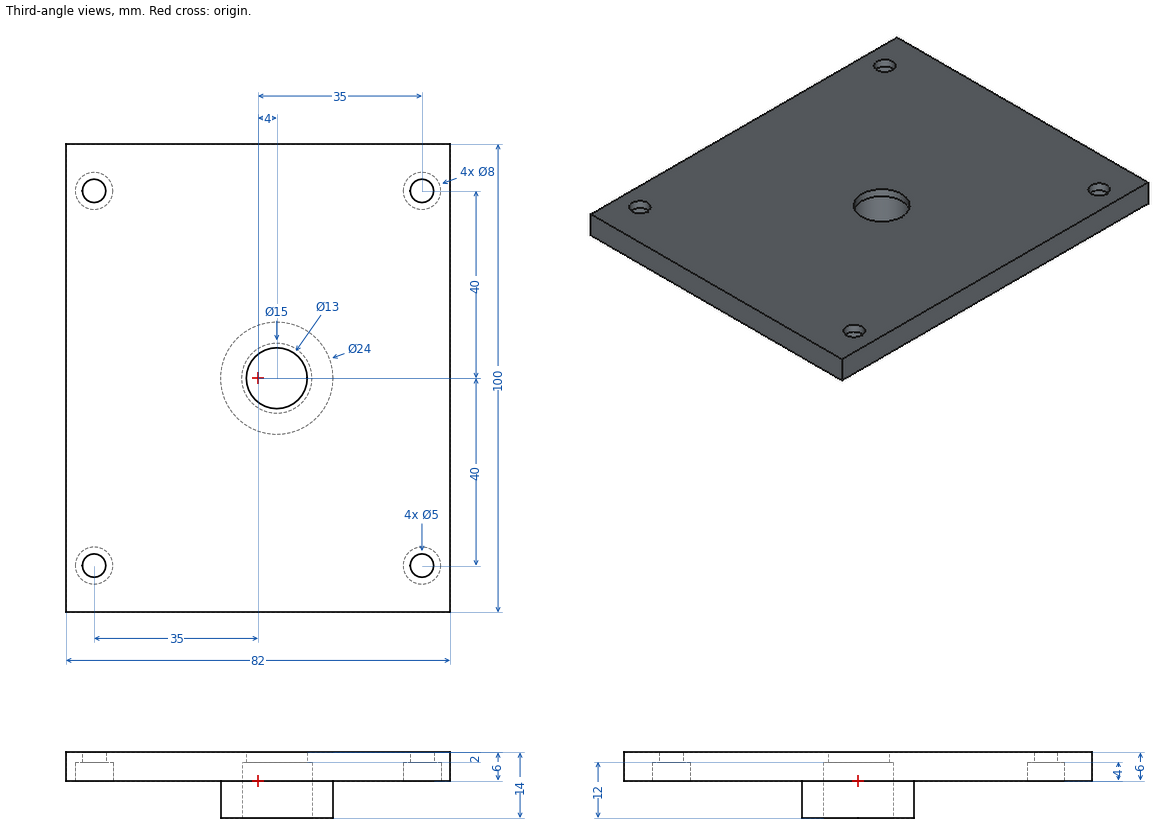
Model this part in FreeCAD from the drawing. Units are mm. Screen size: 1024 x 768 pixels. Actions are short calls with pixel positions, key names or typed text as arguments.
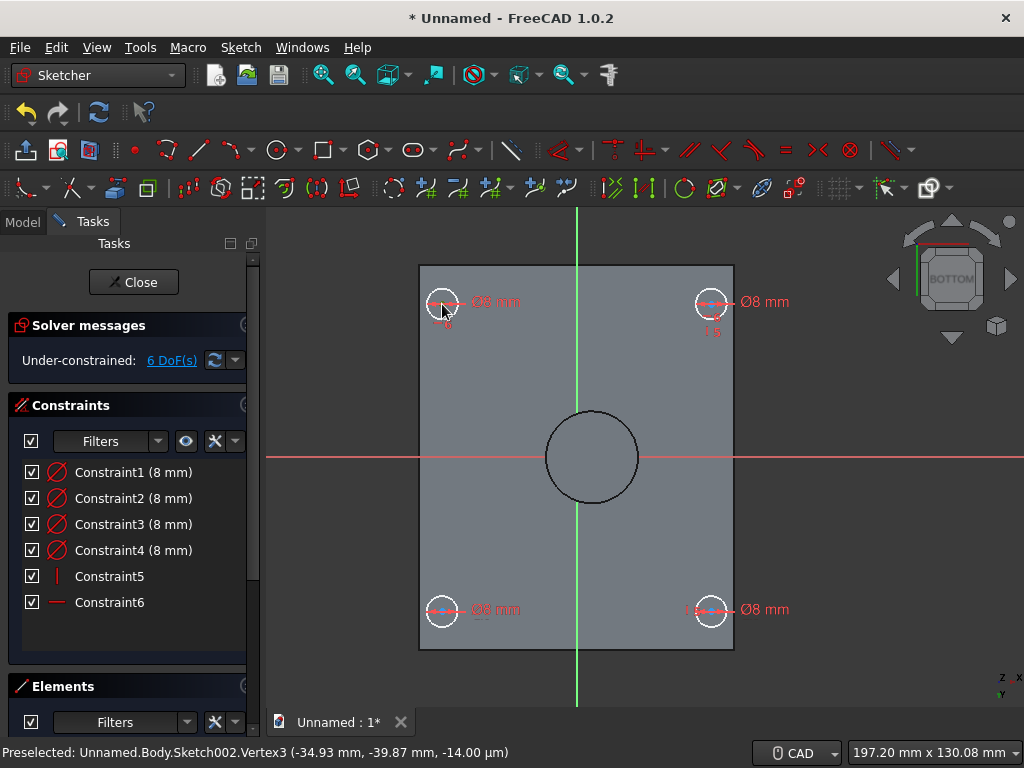
click(442, 612)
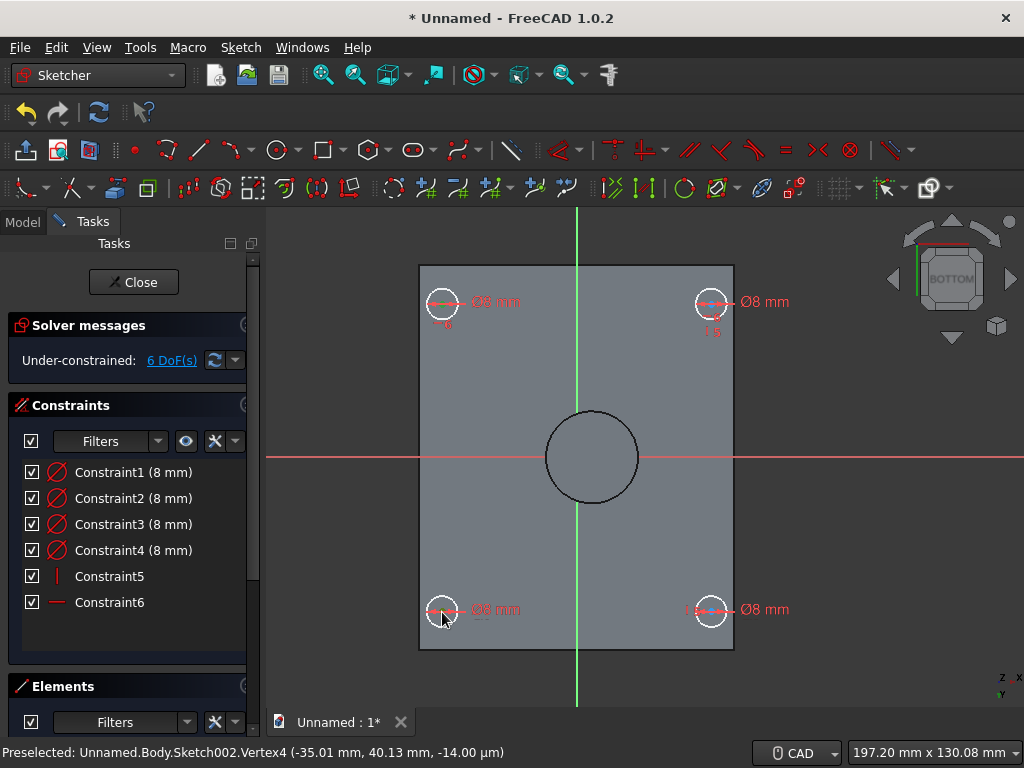
click(668, 150)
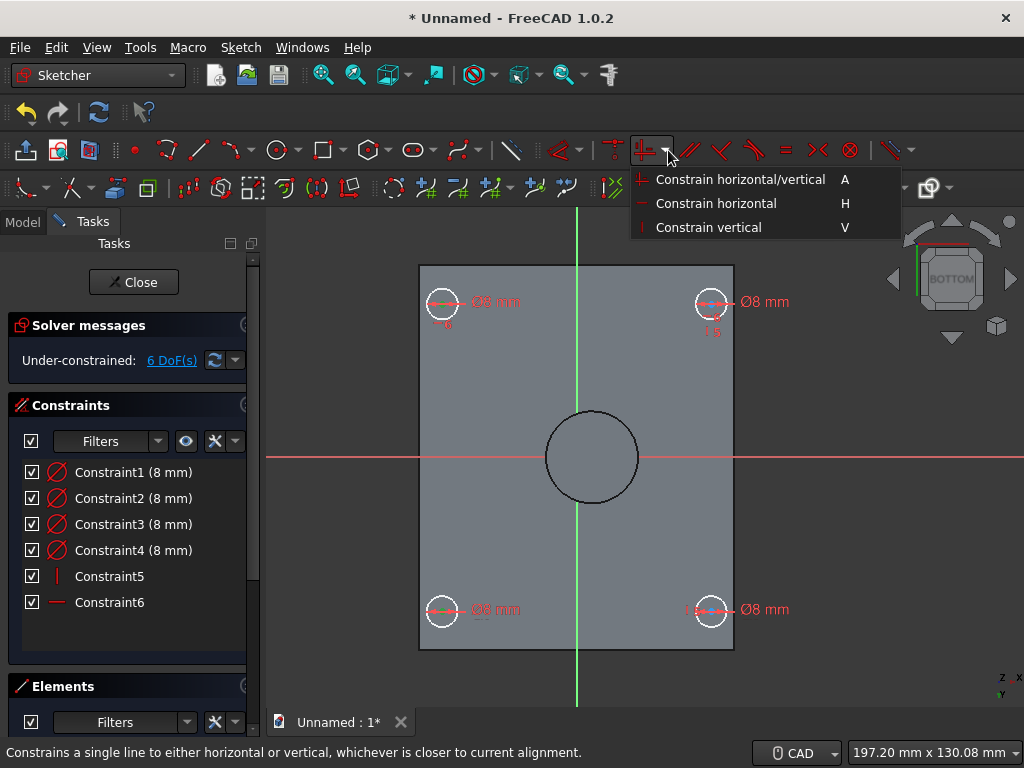
click(766, 227)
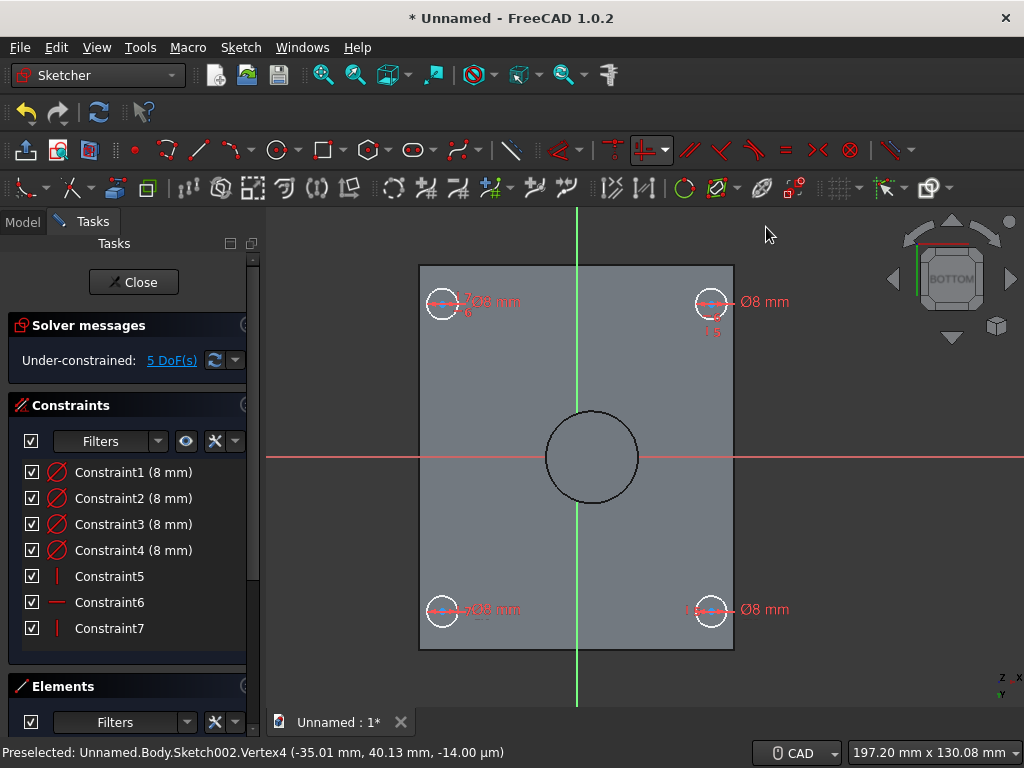
click(711, 612)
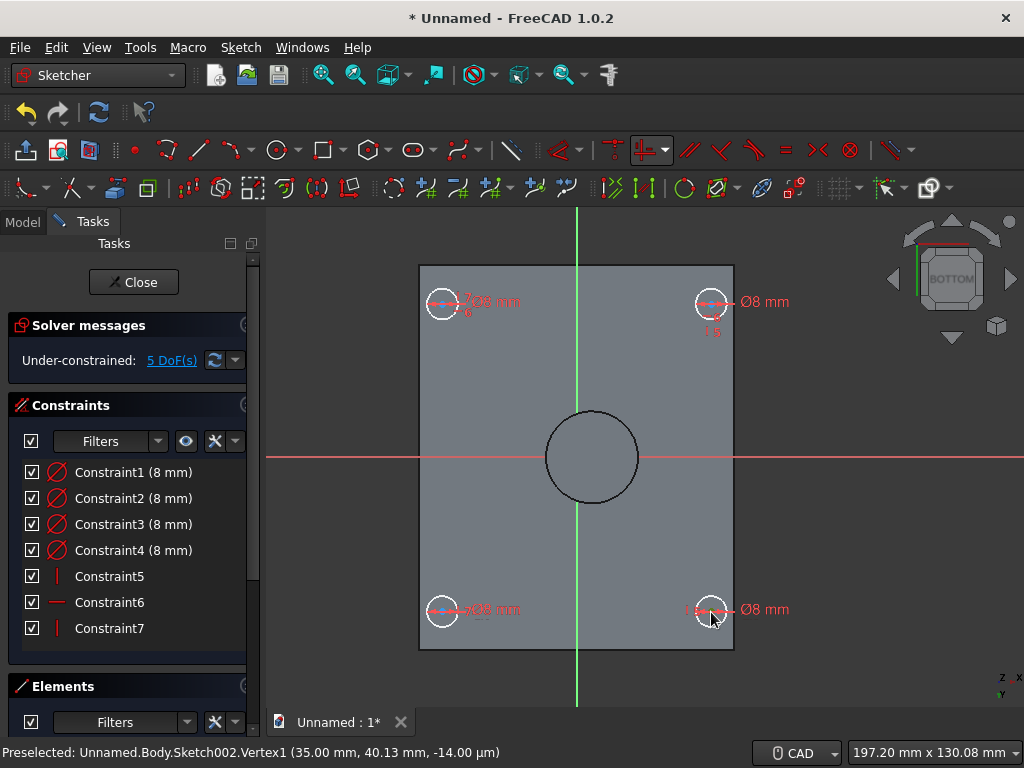
click(442, 612)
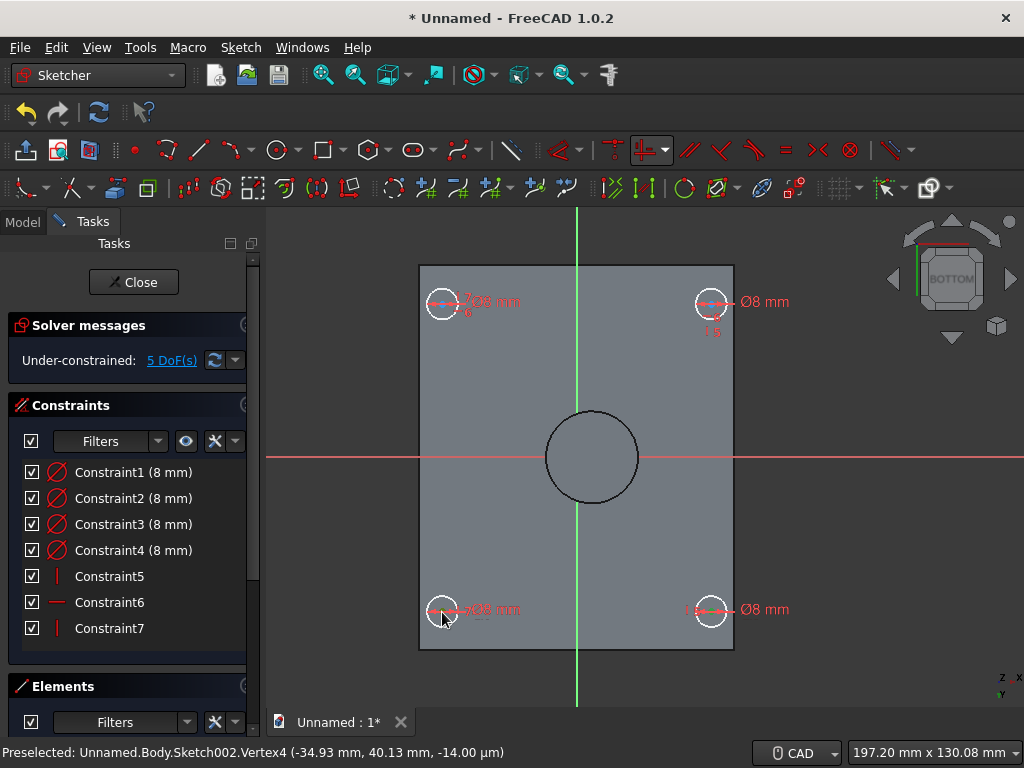
key(h)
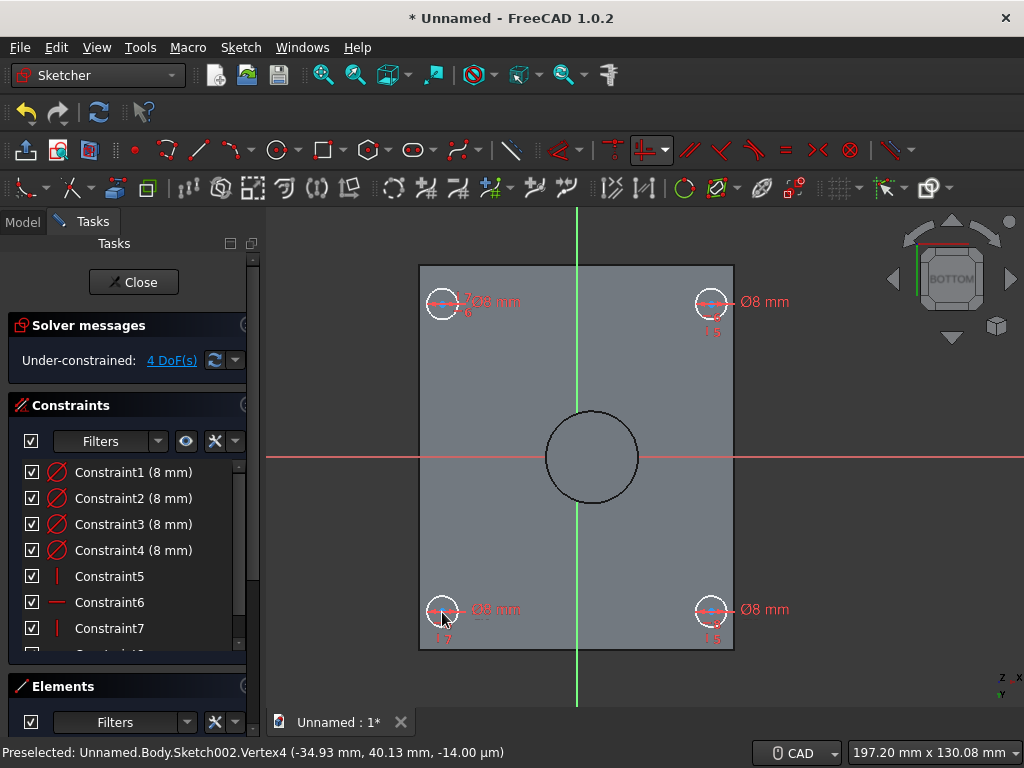
click(711, 612)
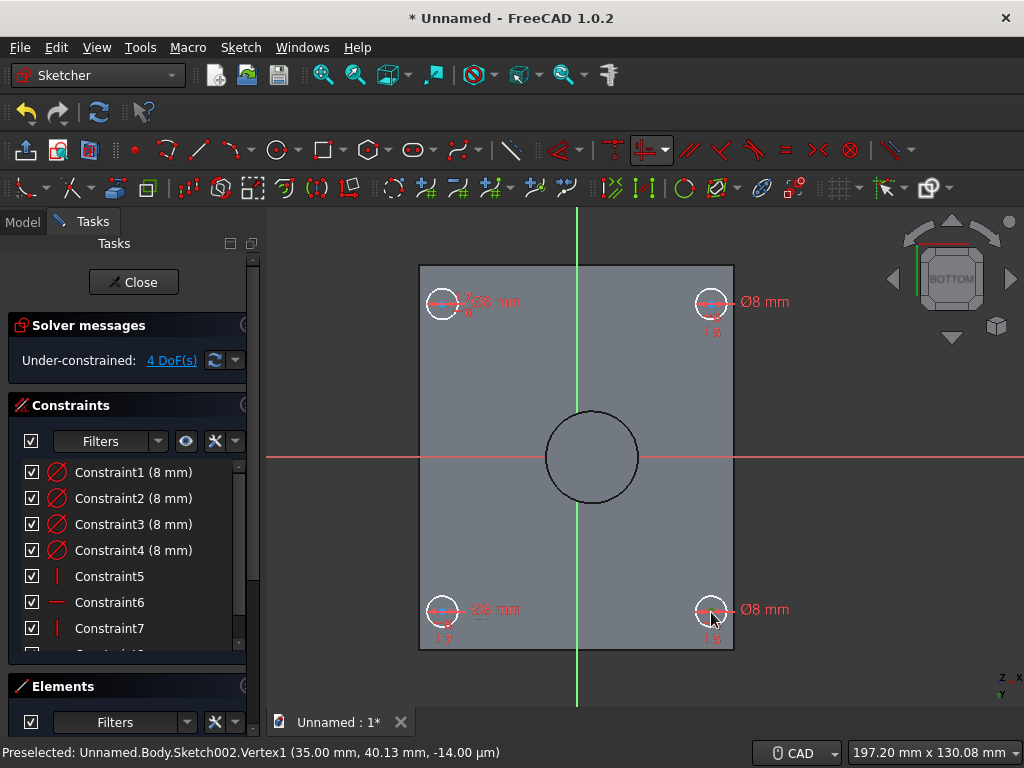
key(l)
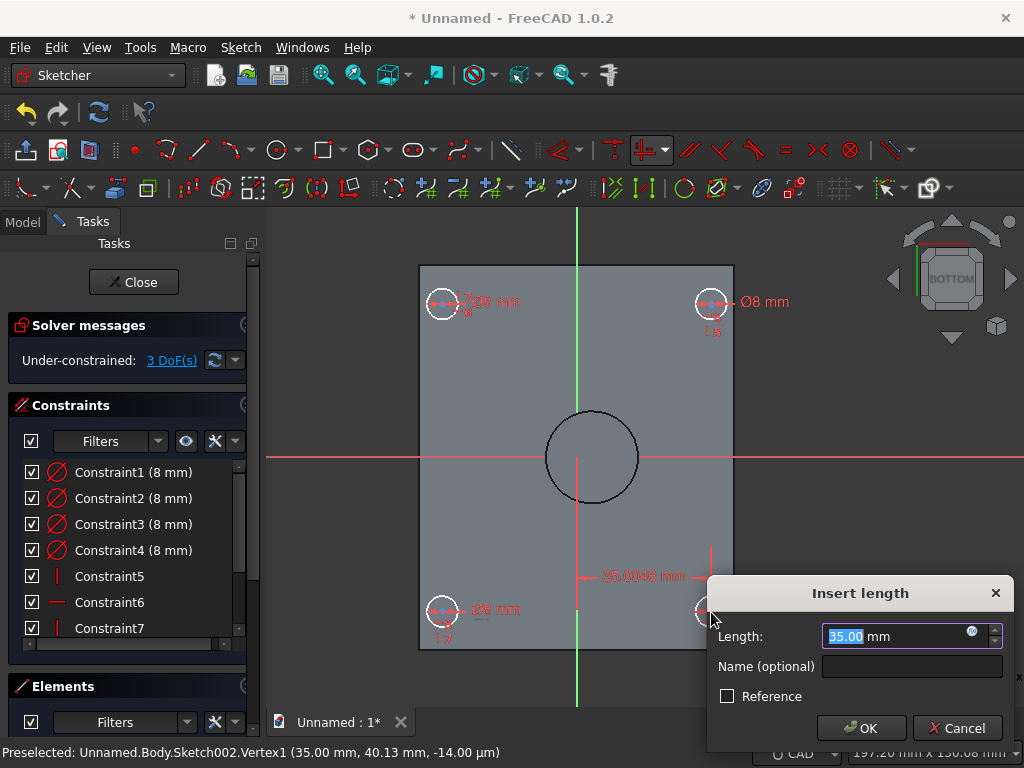
text(35)
key(Return)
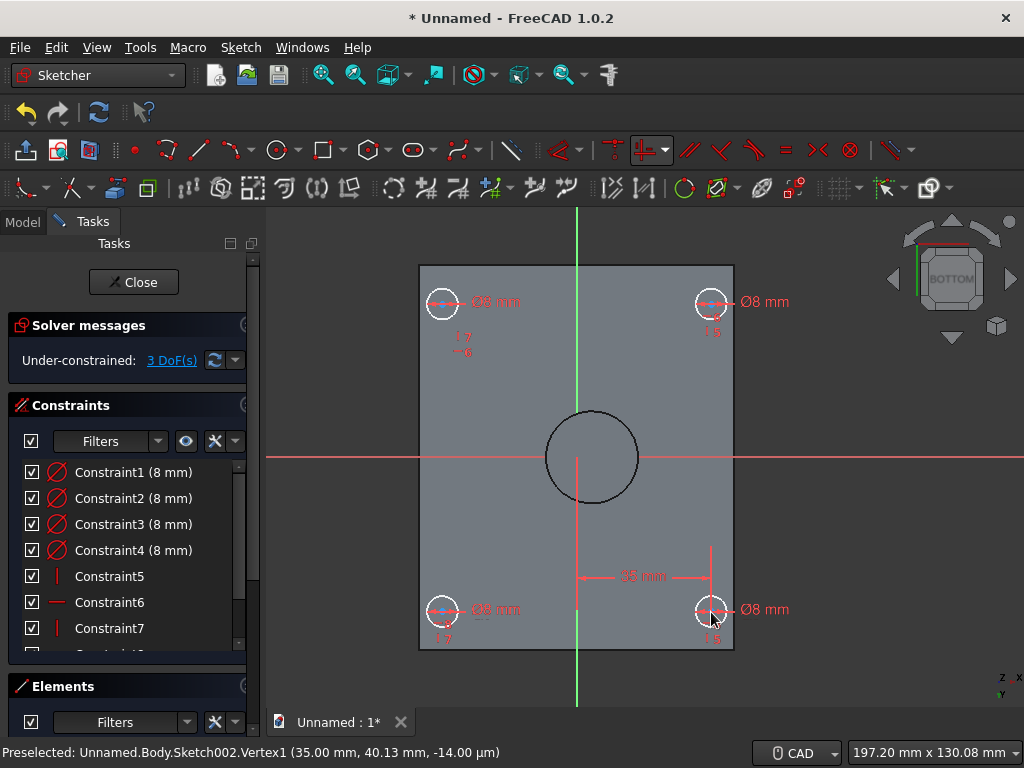
click(711, 612)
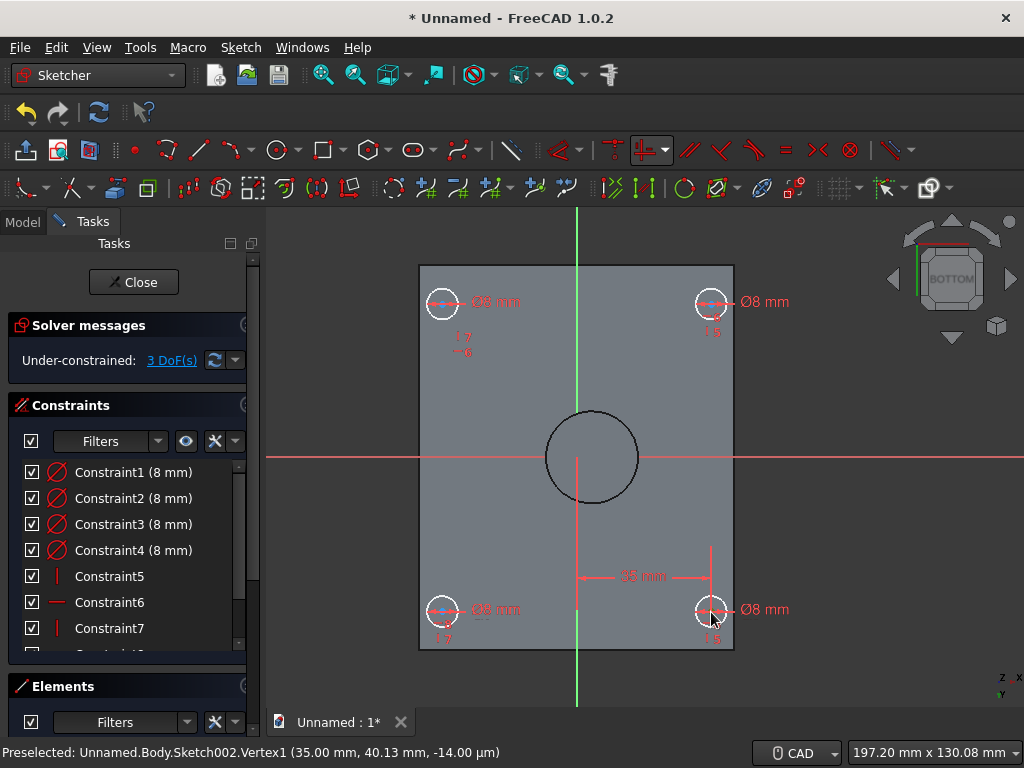
key(i)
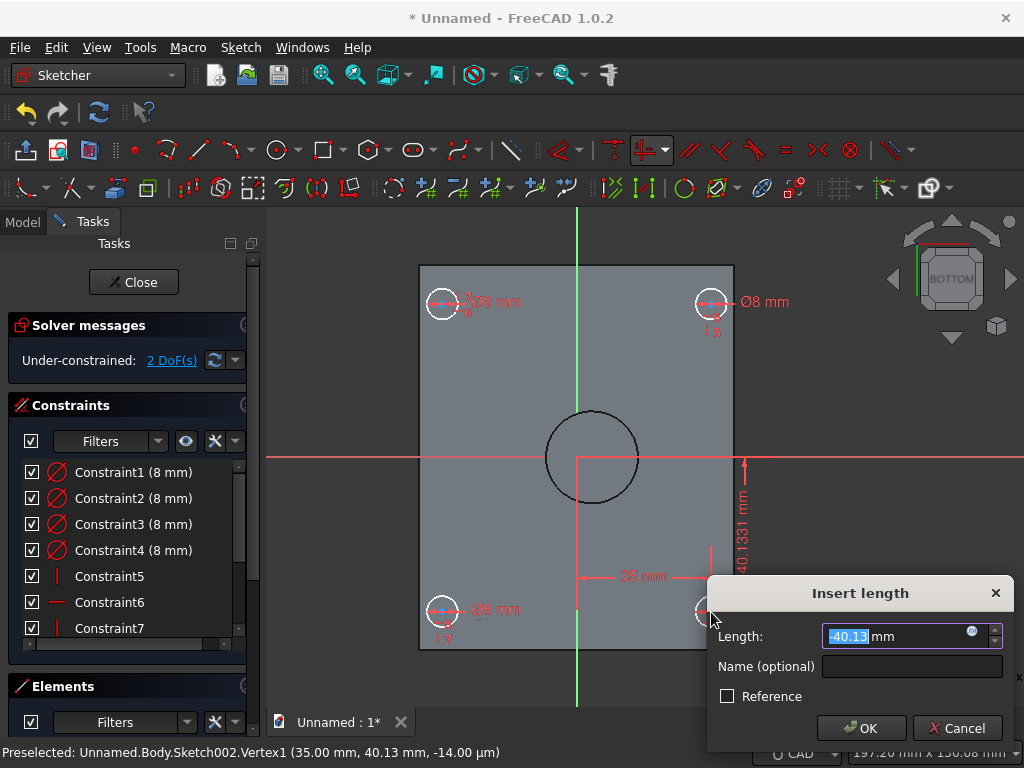
text(-40)
key(Return)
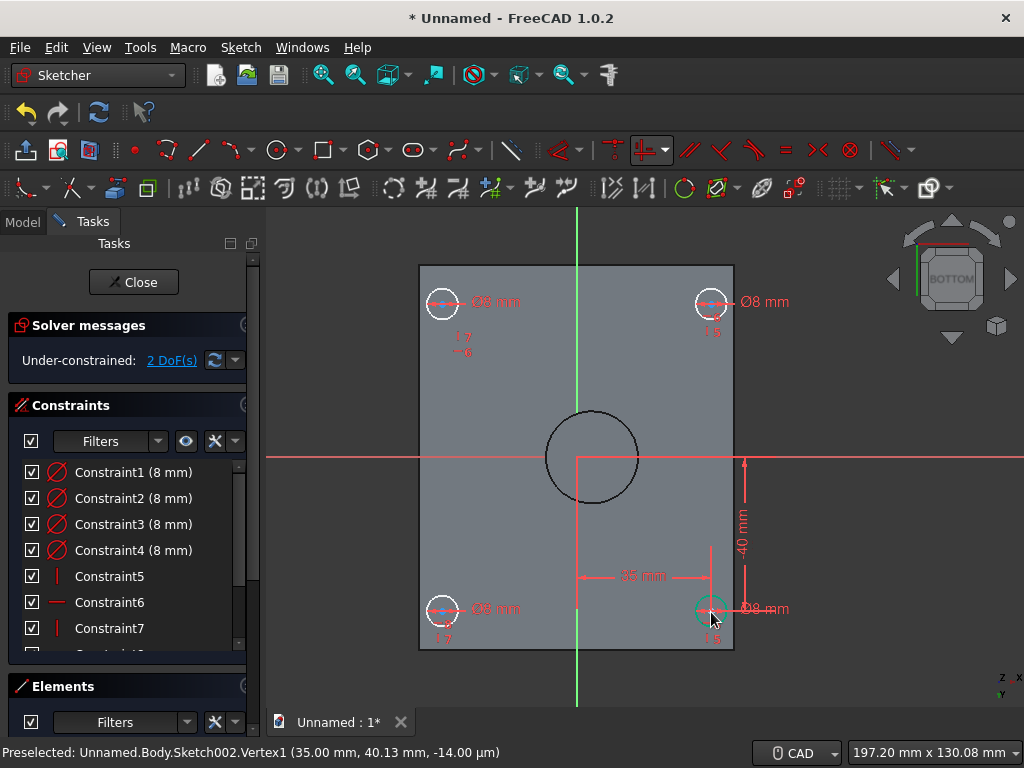
click(711, 304)